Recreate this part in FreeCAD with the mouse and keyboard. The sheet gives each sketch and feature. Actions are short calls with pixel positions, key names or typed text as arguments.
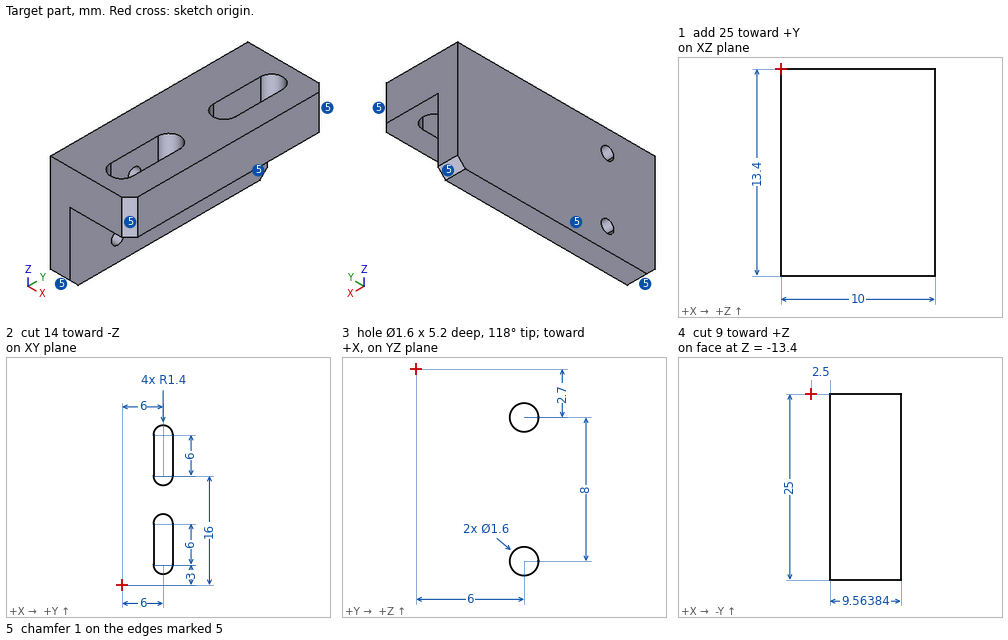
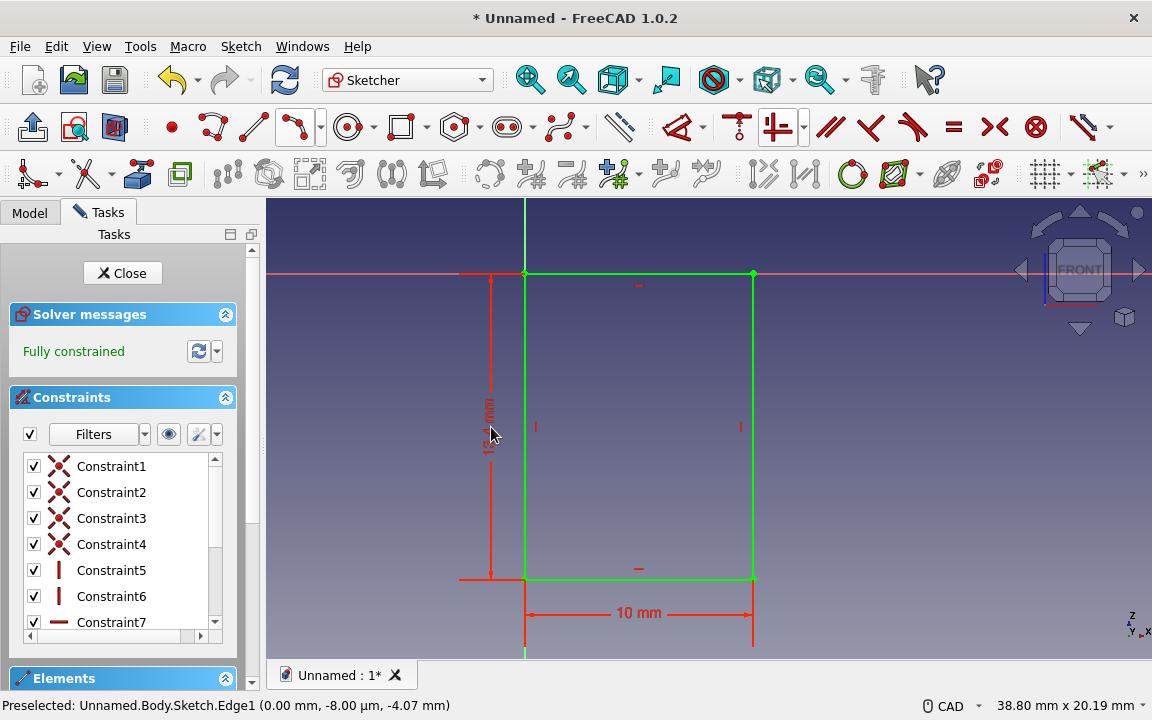
click(123, 273)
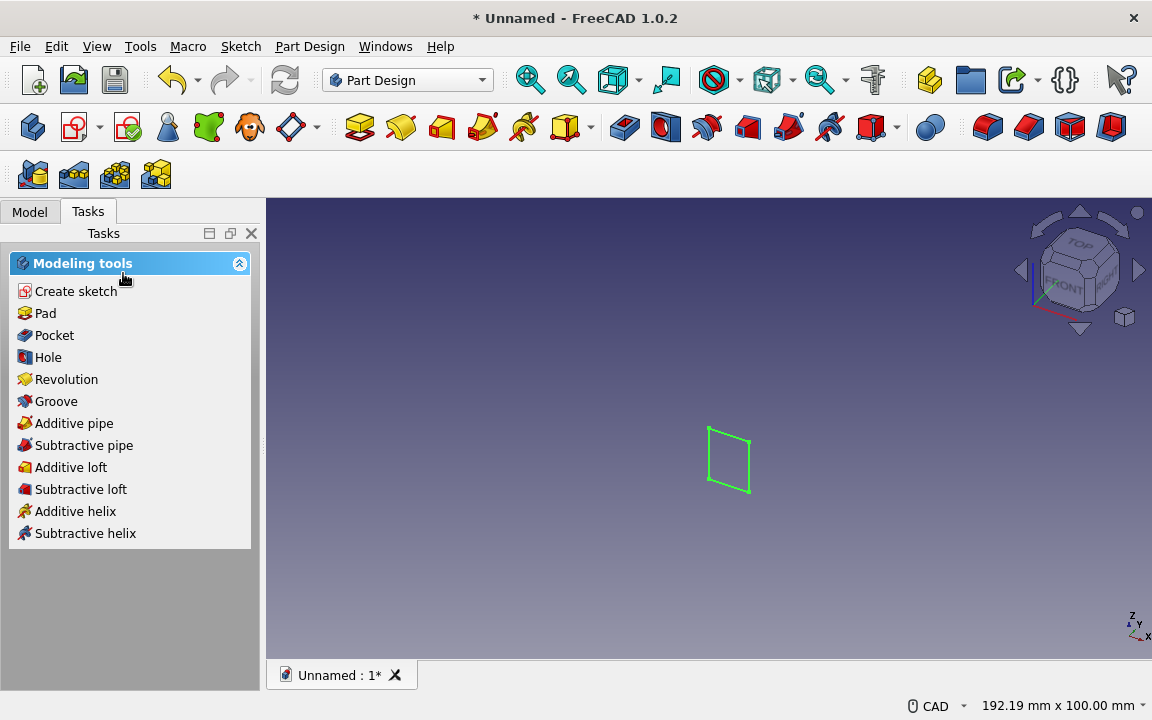
click(360, 128)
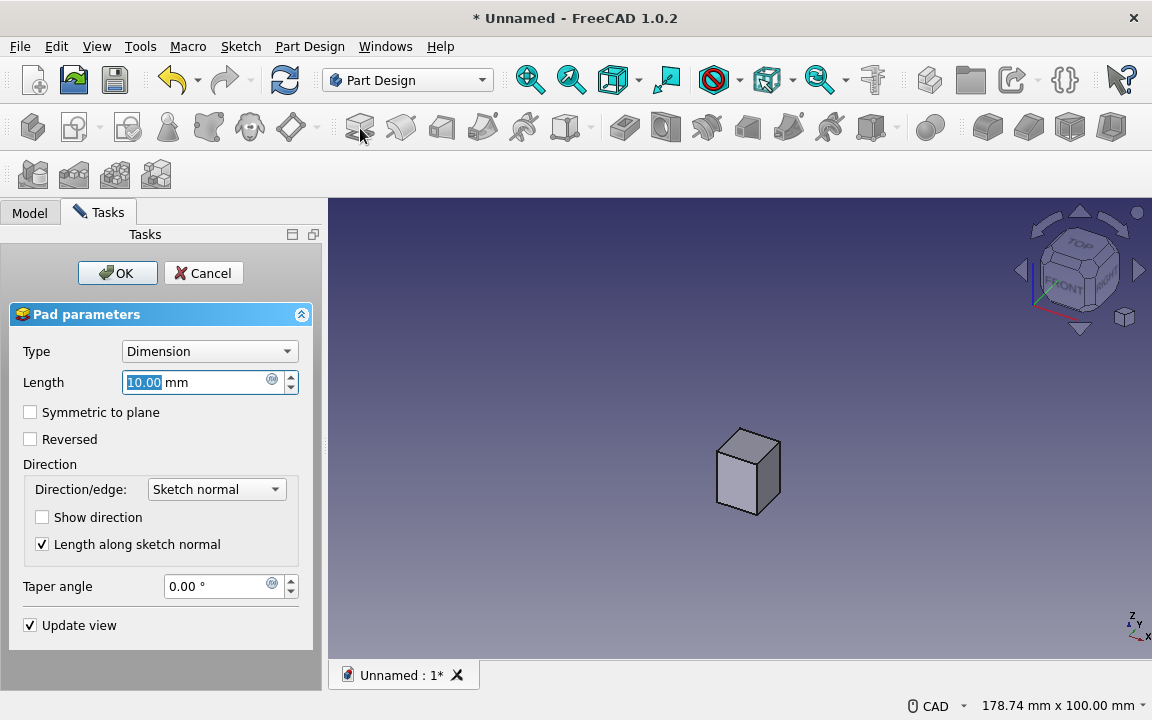
text(25)
key(Tab)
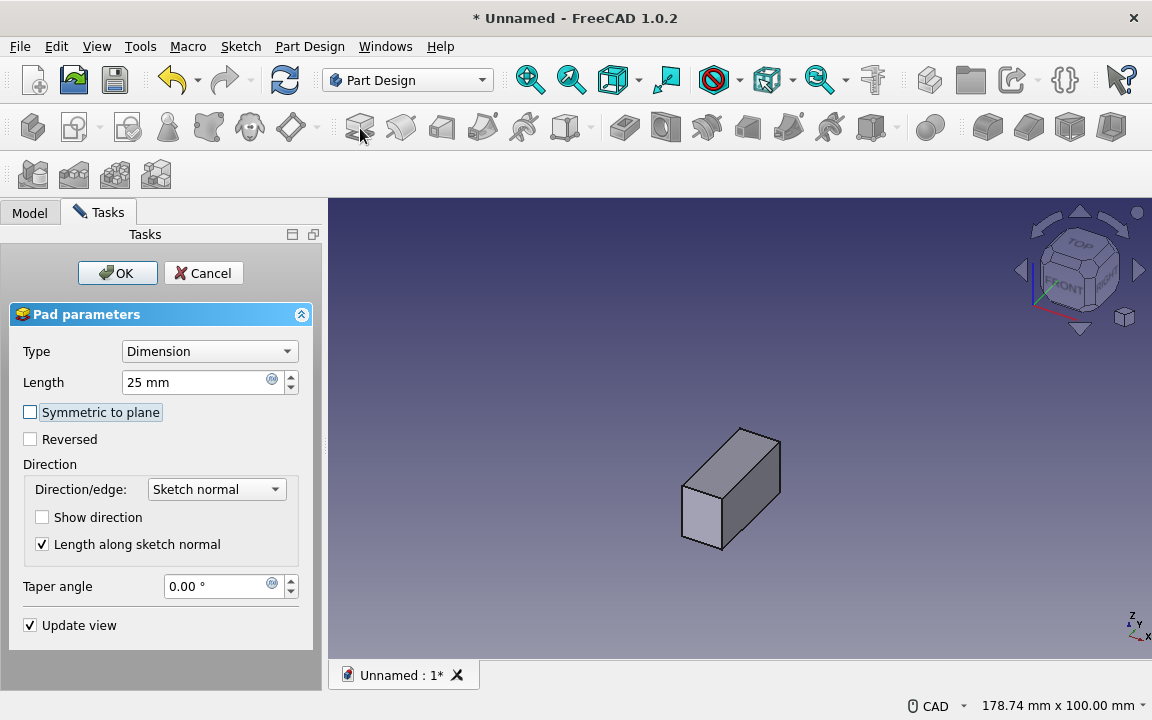
click(31, 439)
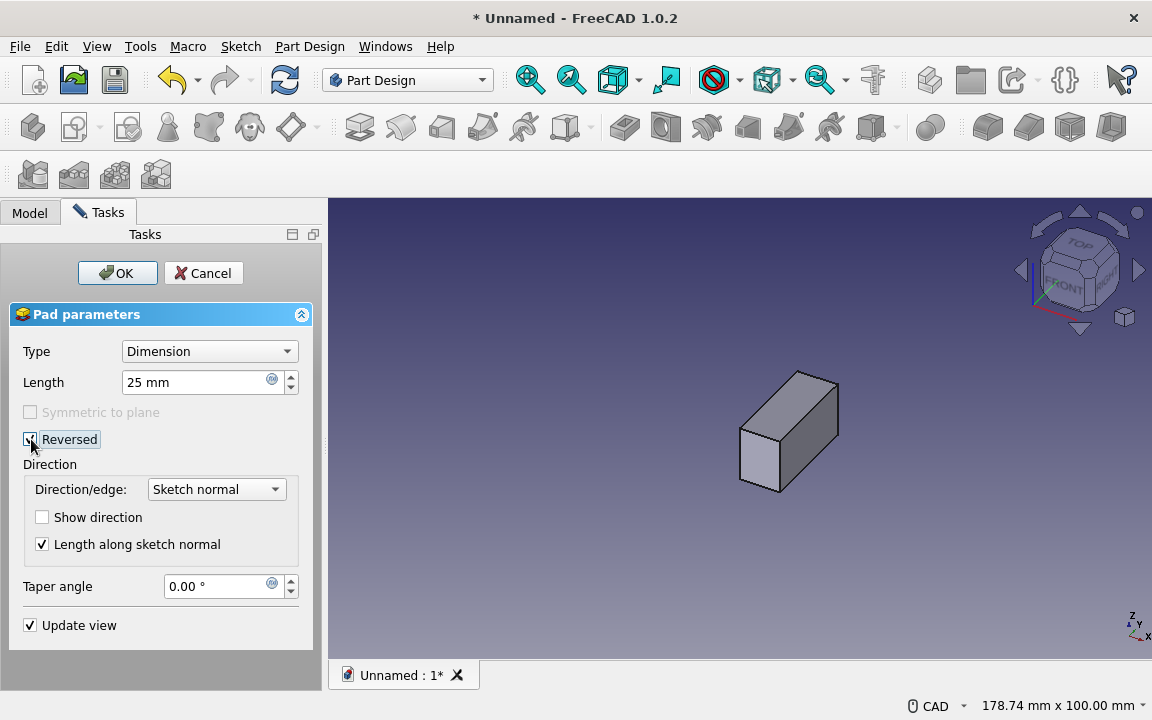
click(118, 273)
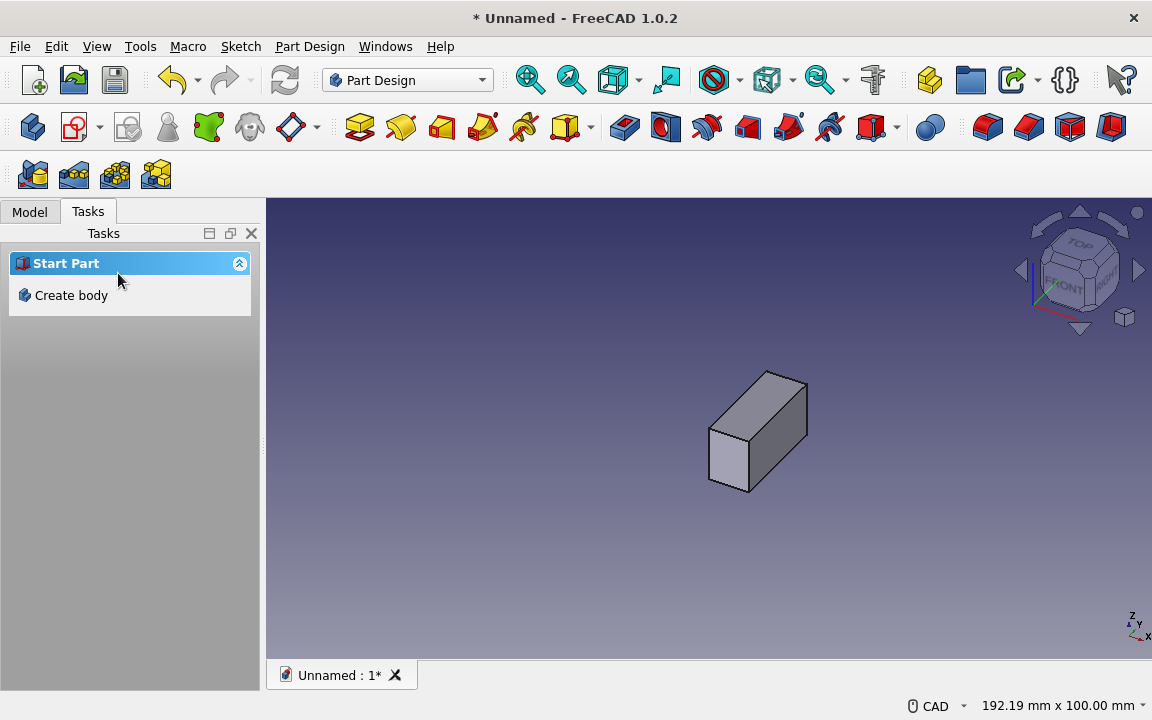
click(531, 80)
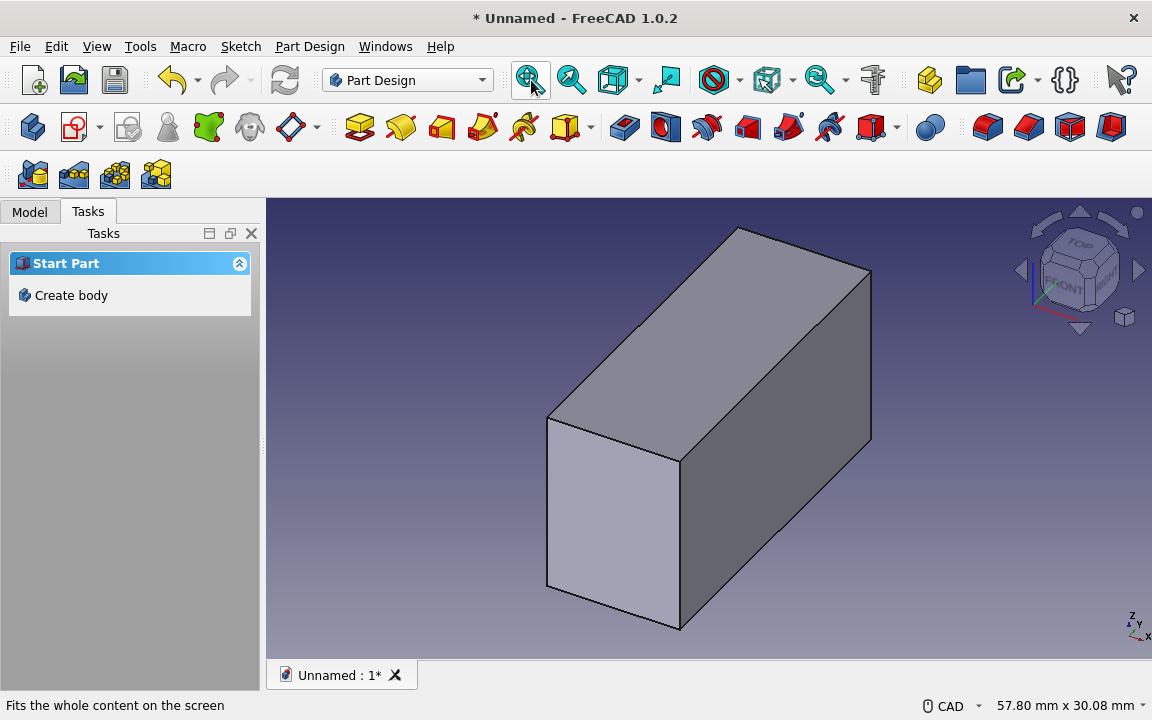
click(74, 128)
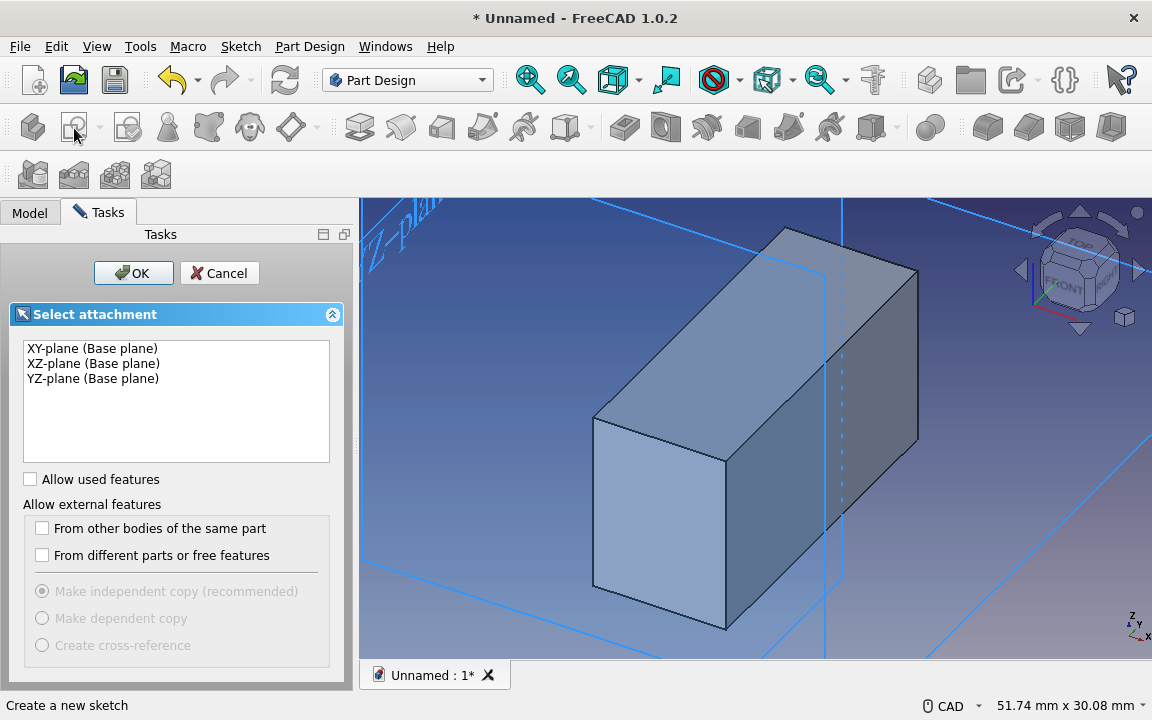
click(84, 348)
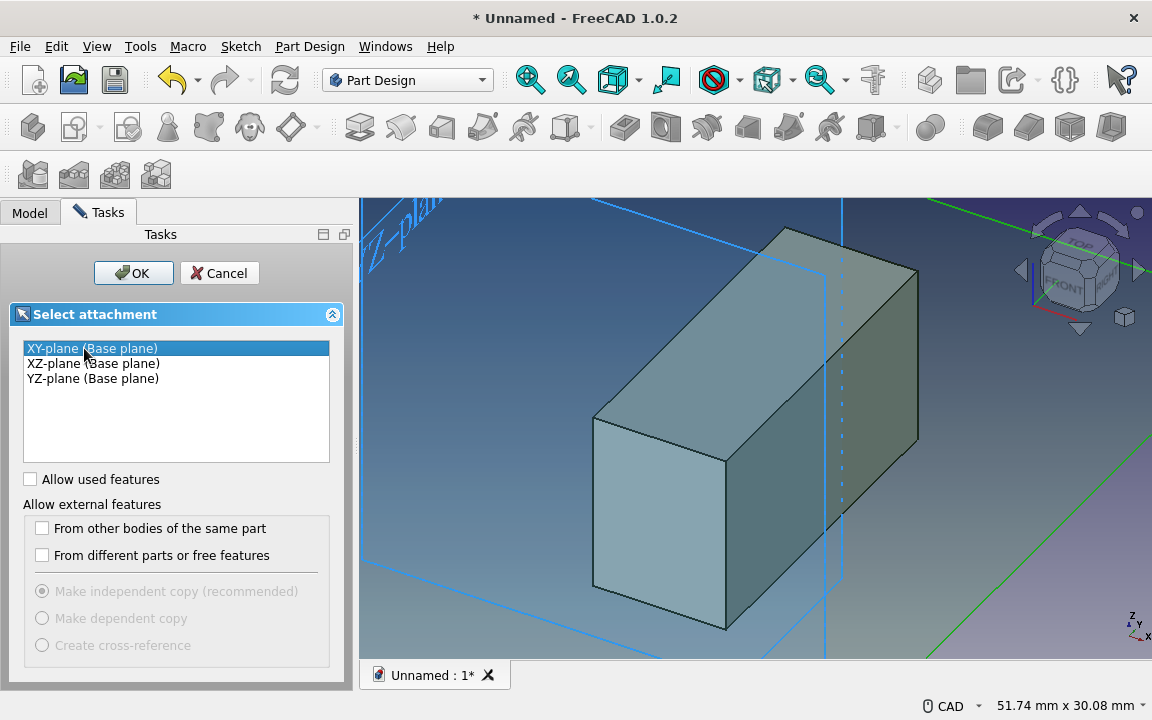
click(134, 273)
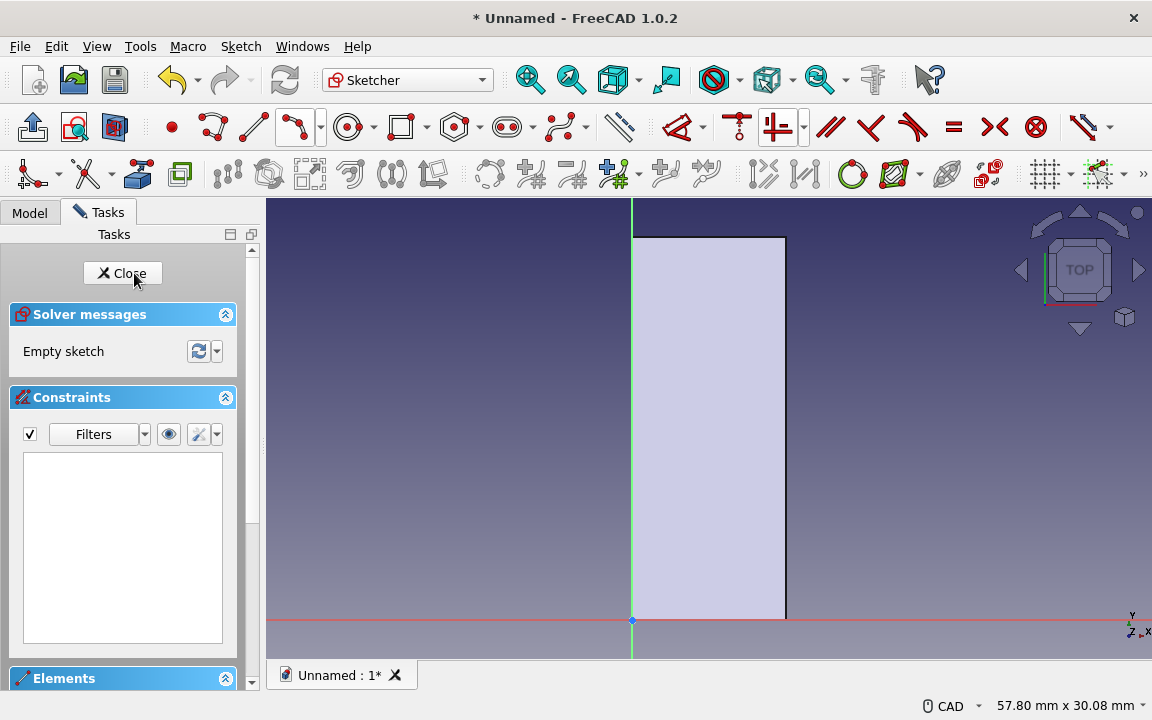
scroll(421, 373, down, 1)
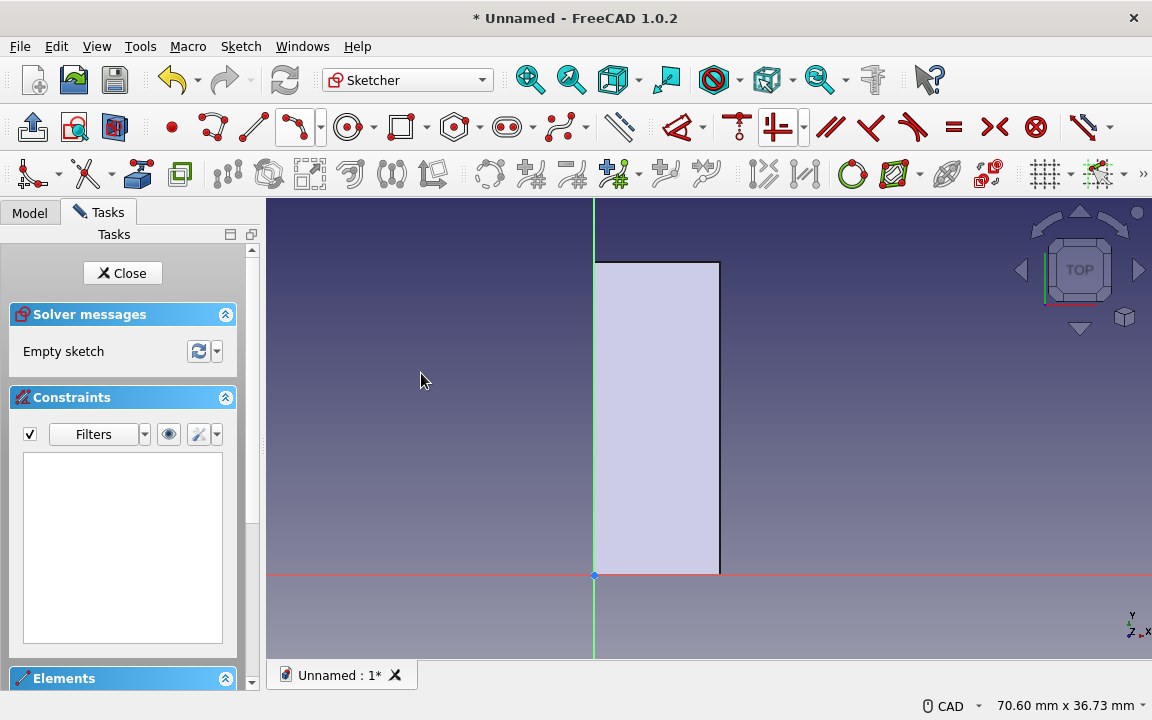
click(506, 128)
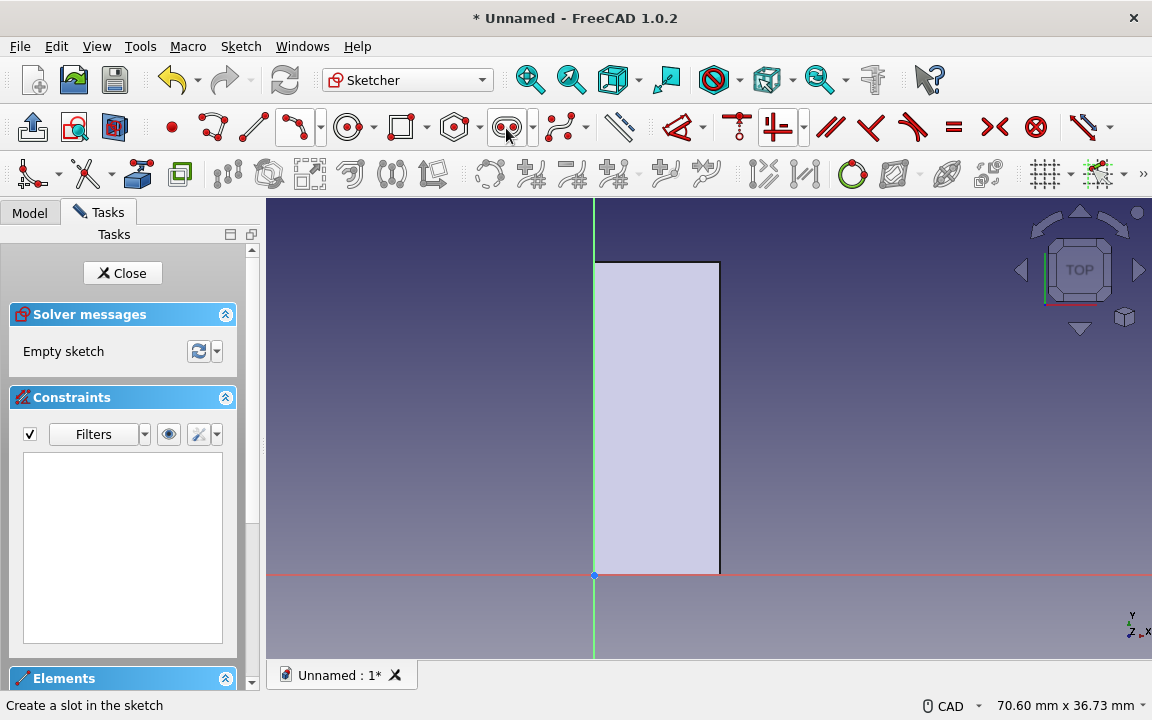
scroll(669, 375, up, 2)